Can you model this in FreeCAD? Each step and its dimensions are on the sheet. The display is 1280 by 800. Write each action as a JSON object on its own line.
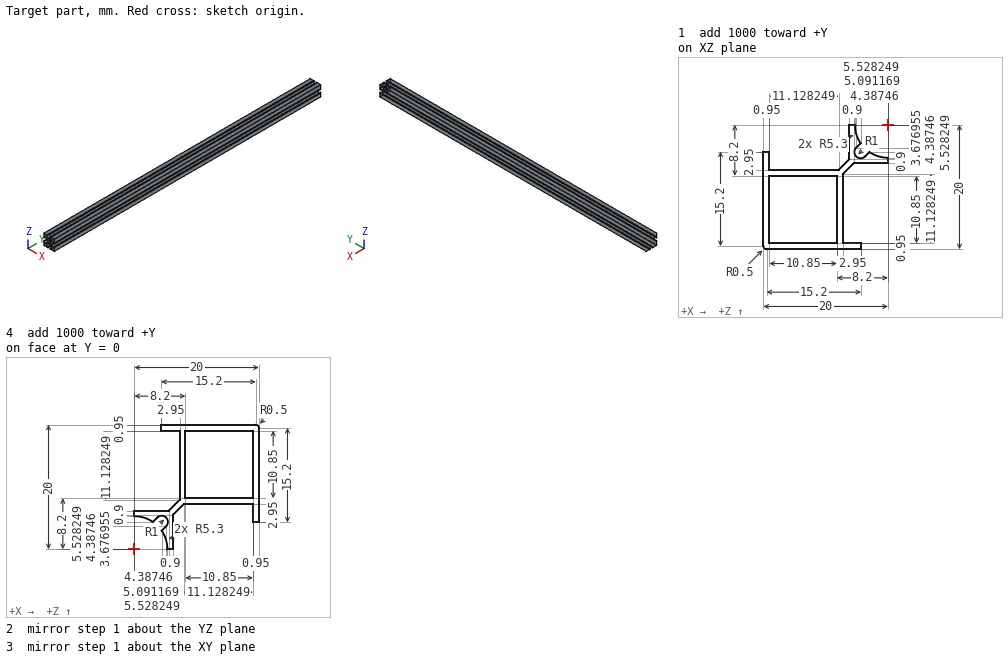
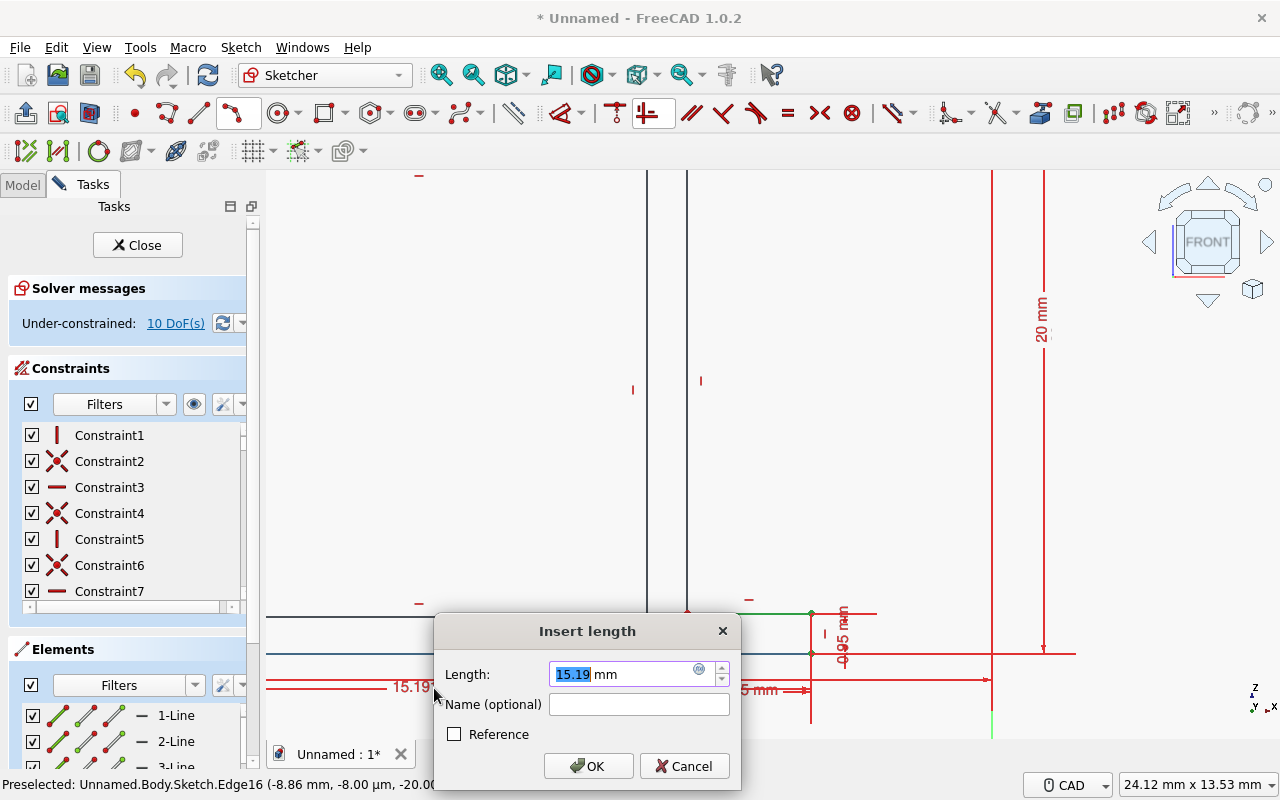
{"action": "type", "text": "15.2"}
{"action": "key", "text": "Return"}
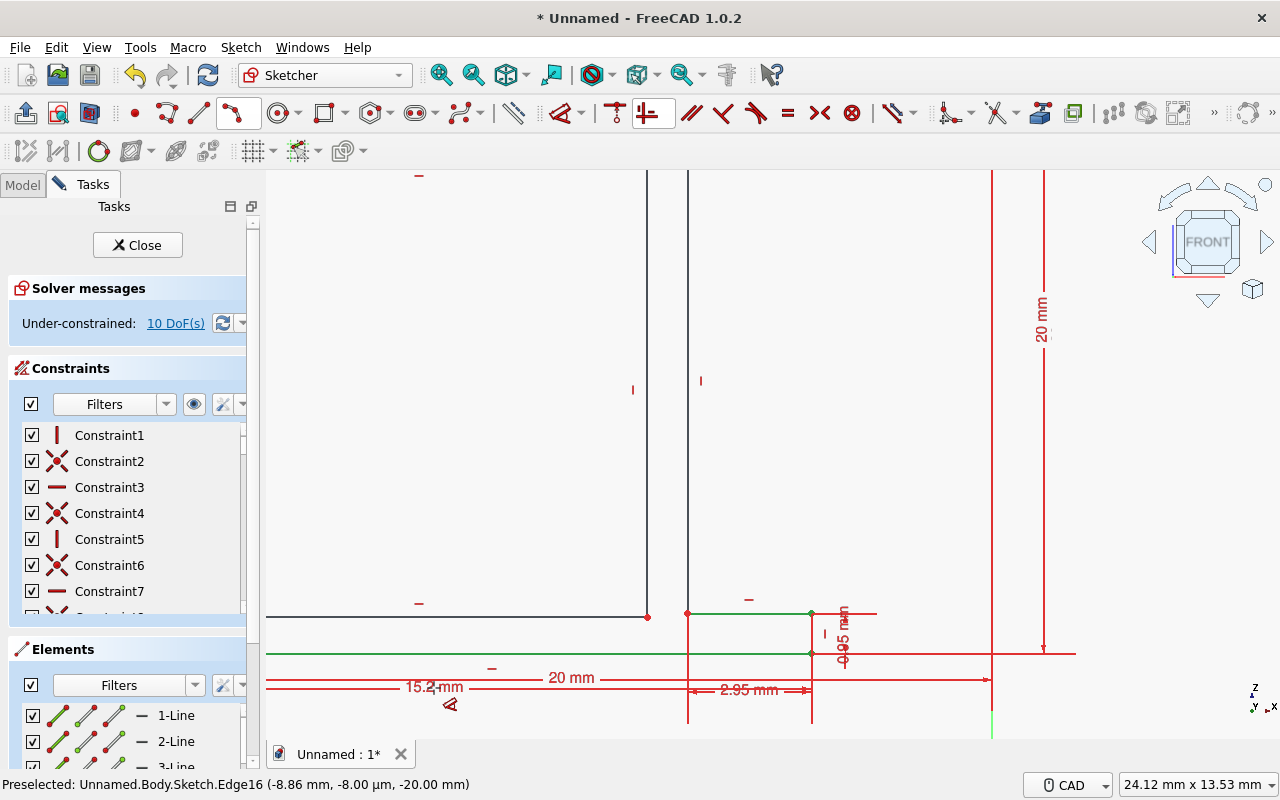
{"action": "scroll", "coordinate": [813, 635], "scroll_direction": "down", "scroll_amount": 4}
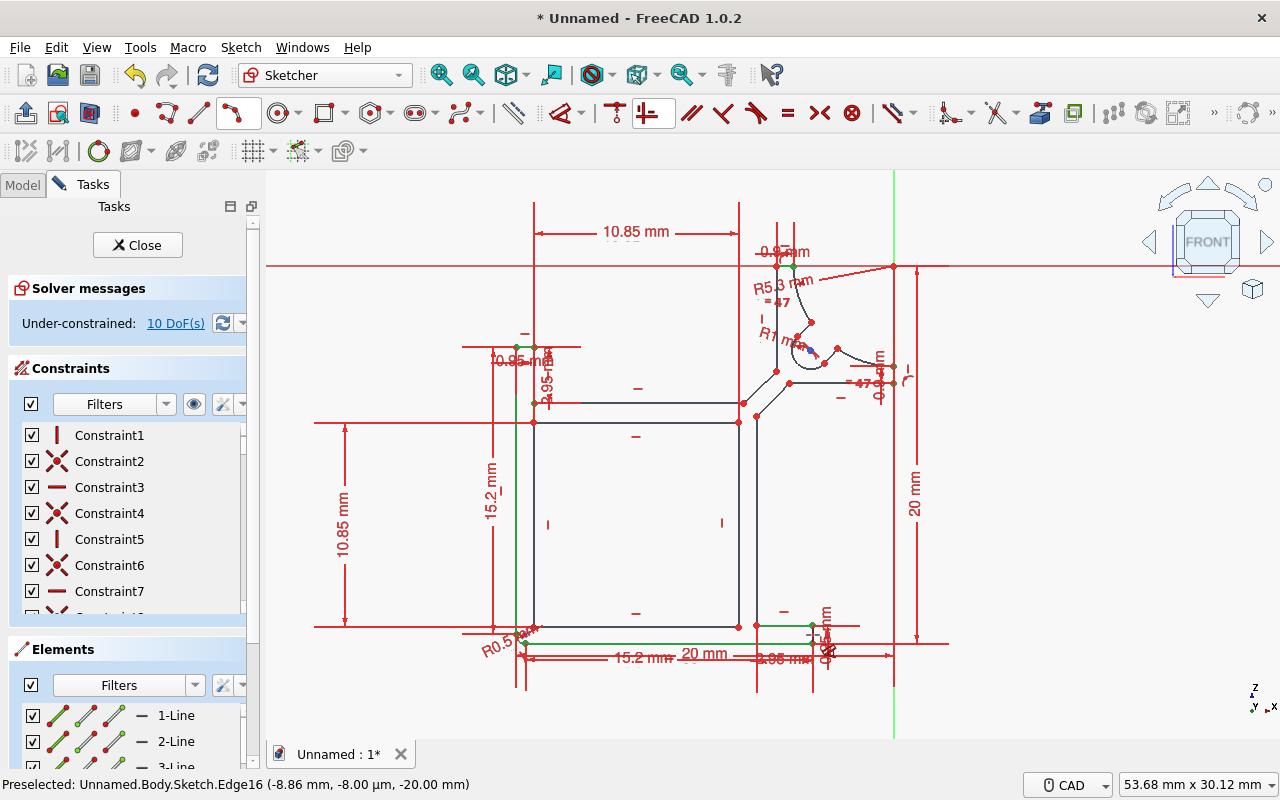
{"action": "left_click", "coordinate": [534, 423]}
{"action": "left_click", "coordinate": [928, 344]}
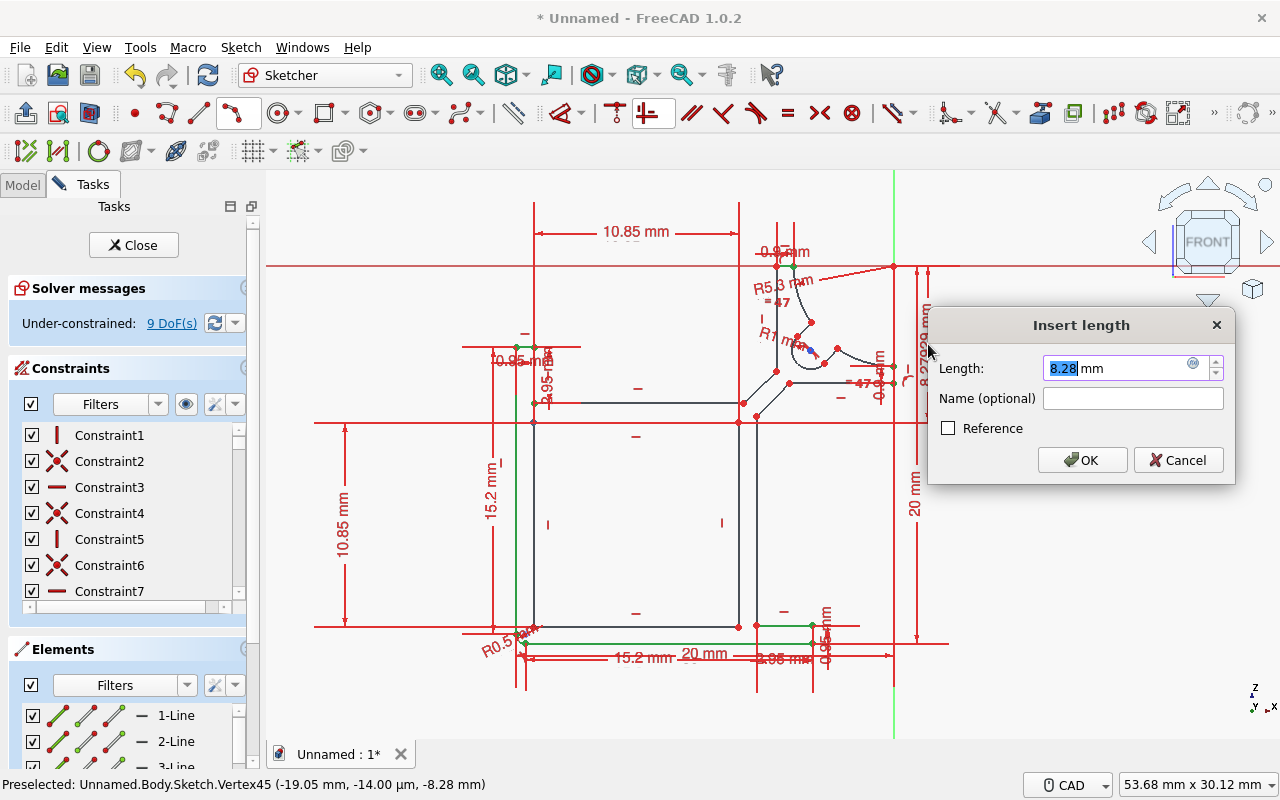
{"action": "type", "text": "8.2"}
{"action": "key", "text": "Return"}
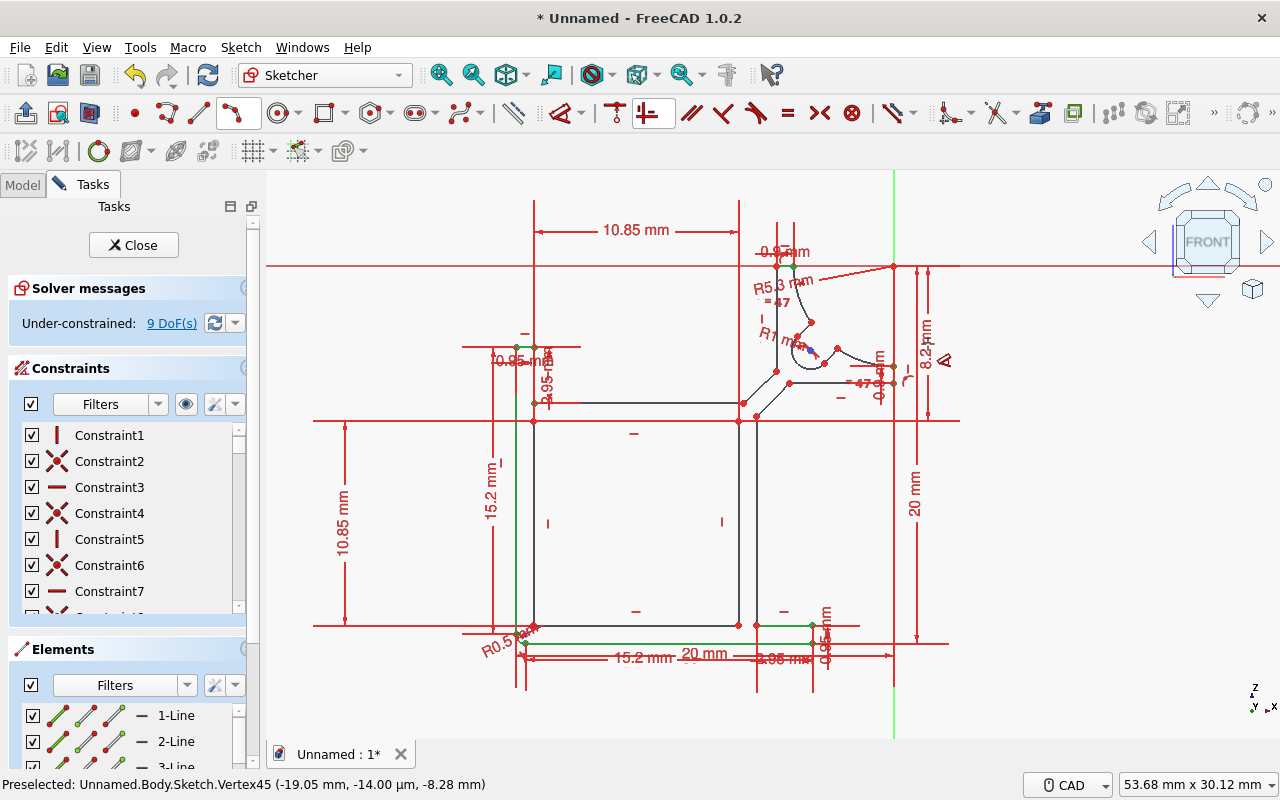
{"action": "left_click", "coordinate": [739, 626]}
{"action": "left_click", "coordinate": [816, 232]}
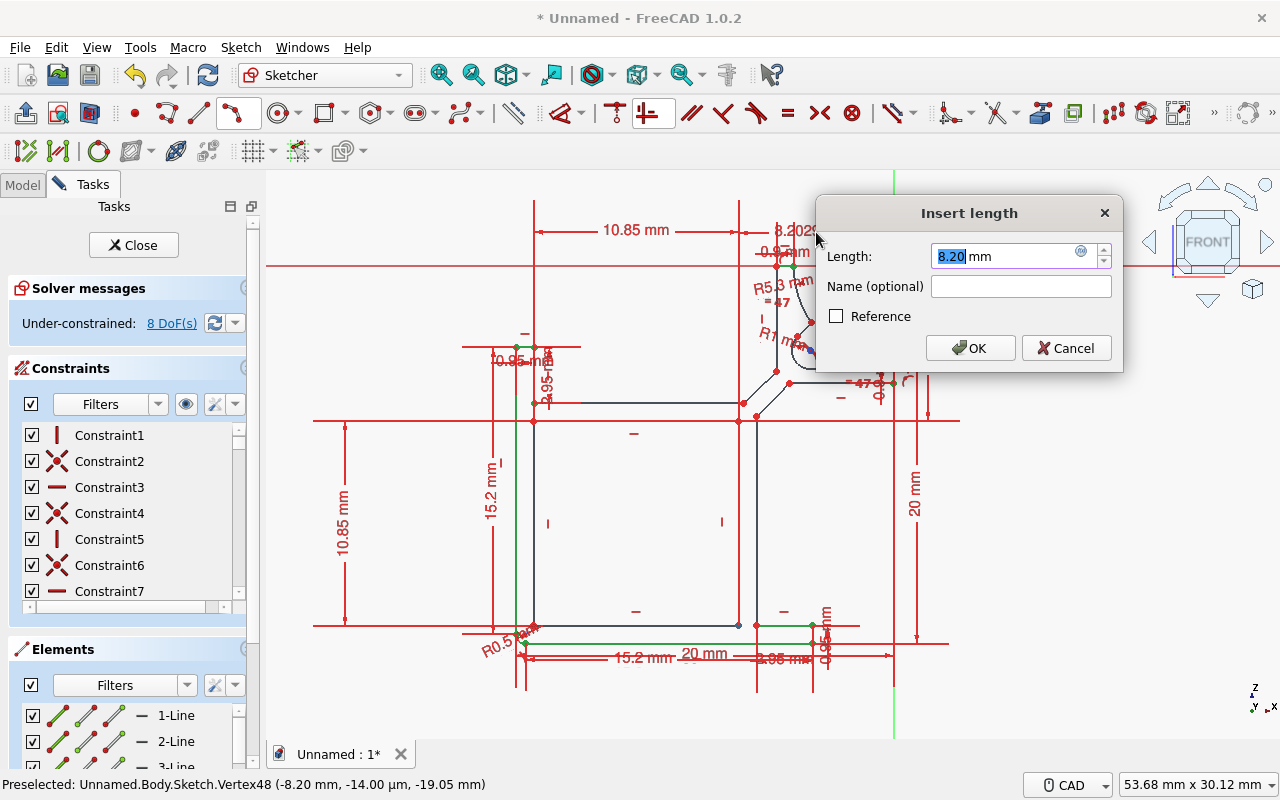
{"action": "type", "text": "8.2"}
{"action": "key", "text": "Return"}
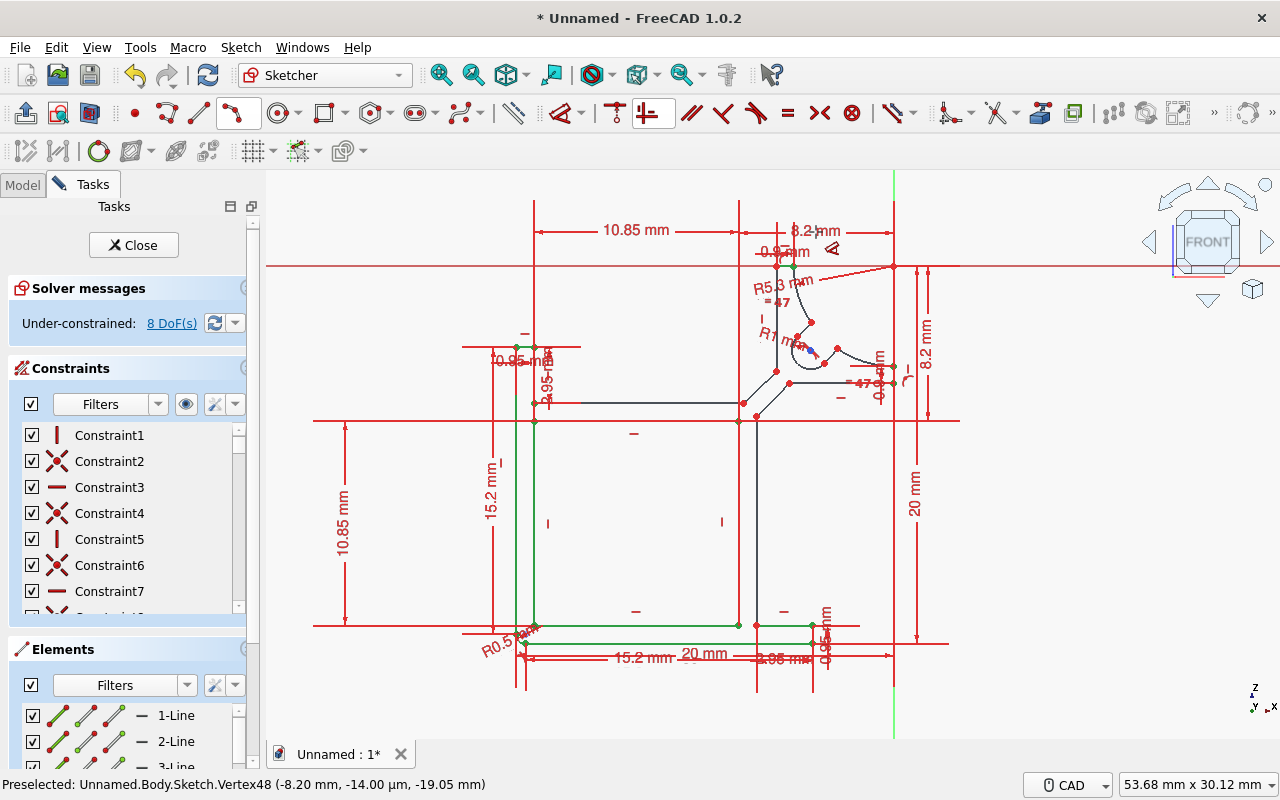
{"action": "left_click", "coordinate": [777, 340]}
{"action": "left_click", "coordinate": [743, 319]}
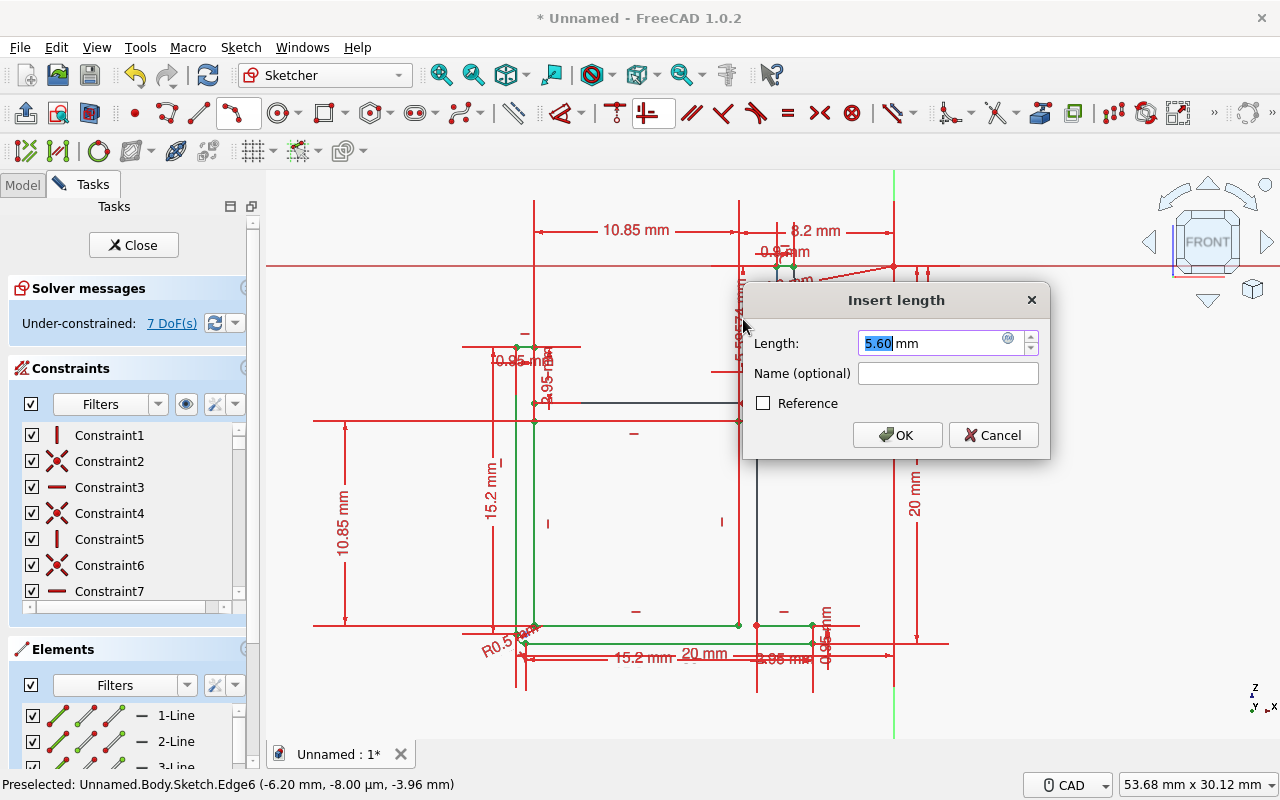
{"action": "type", "text": "5.528249"}
{"action": "key", "text": "Return"}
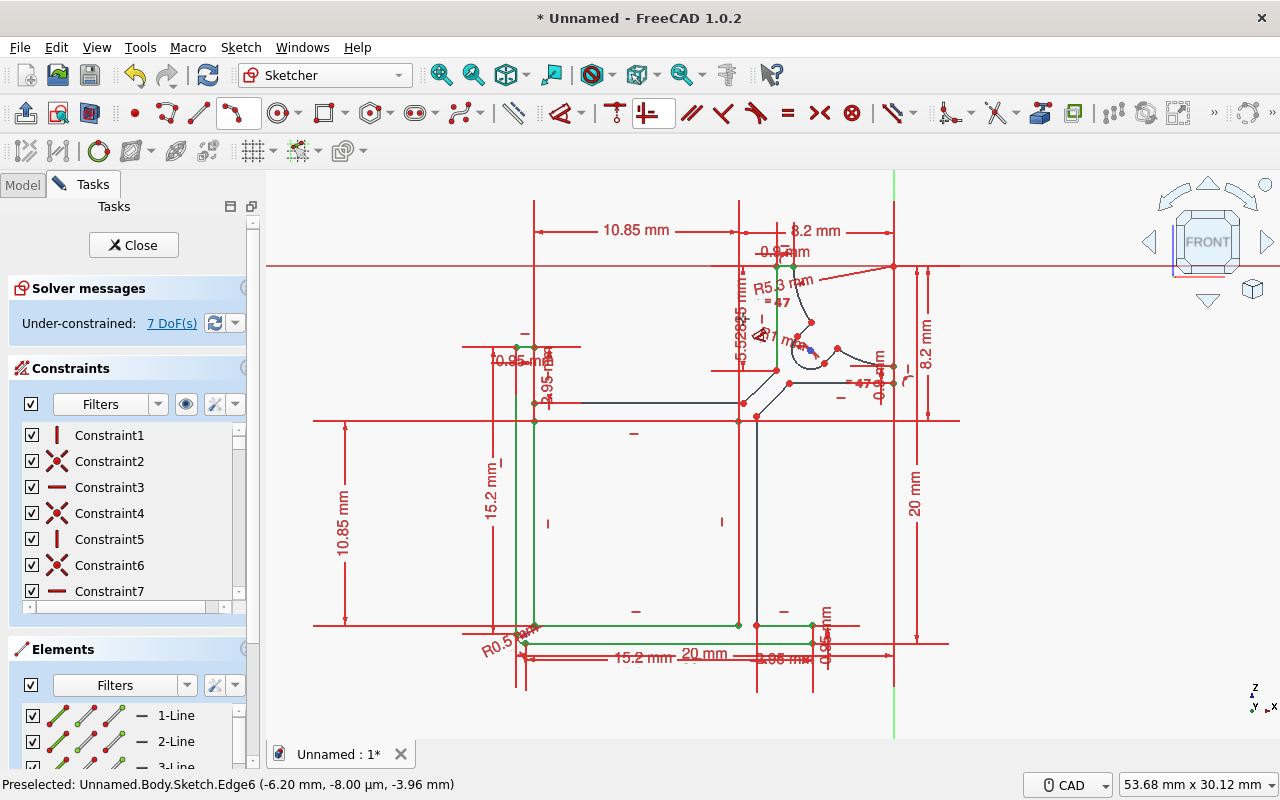
{"action": "left_click", "coordinate": [863, 383]}
{"action": "left_click", "coordinate": [842, 417]}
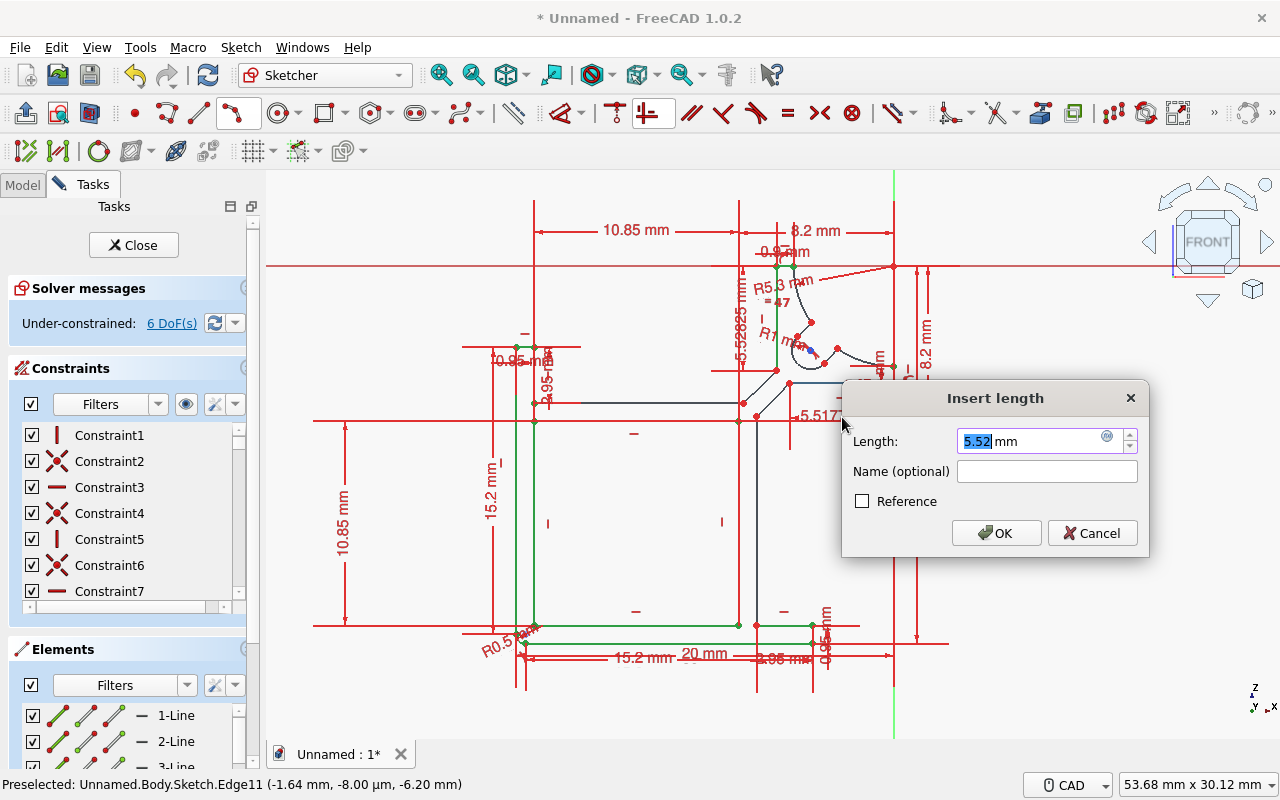
{"action": "type", "text": "5.528249"}
{"action": "key", "text": "Return"}